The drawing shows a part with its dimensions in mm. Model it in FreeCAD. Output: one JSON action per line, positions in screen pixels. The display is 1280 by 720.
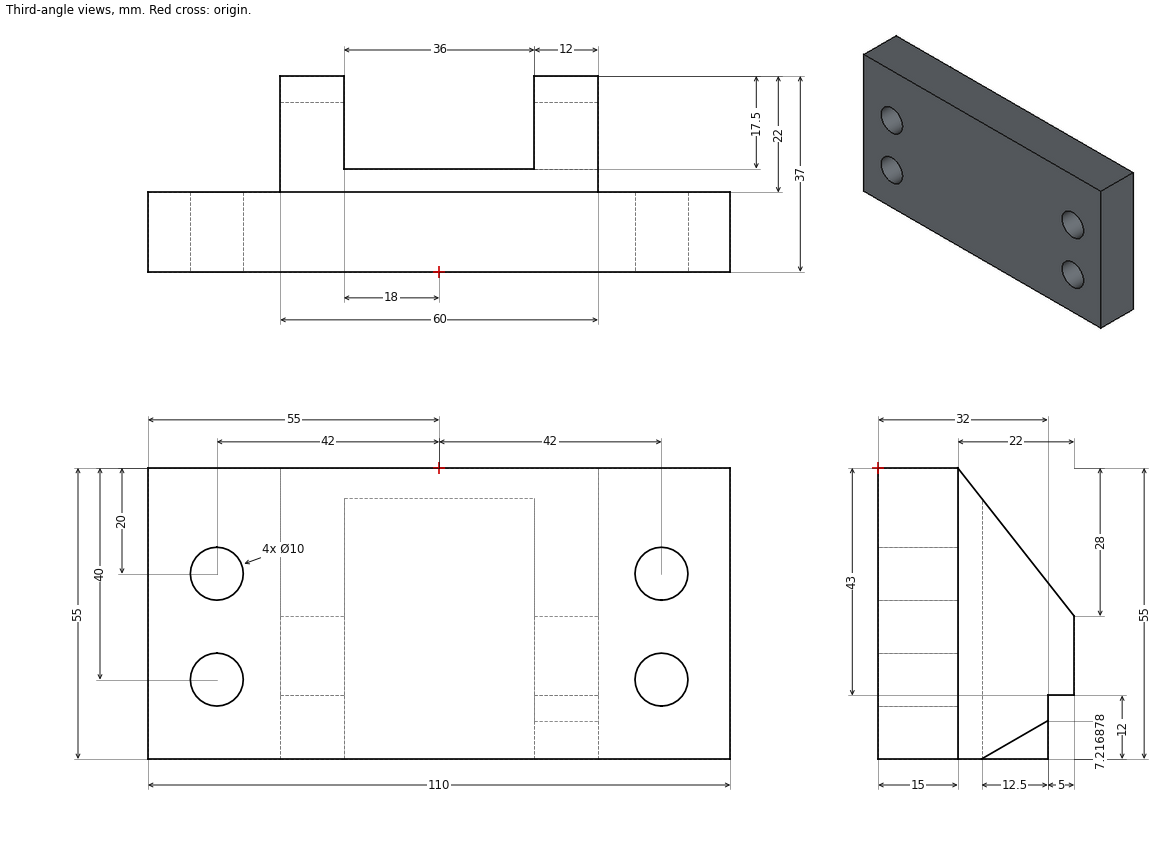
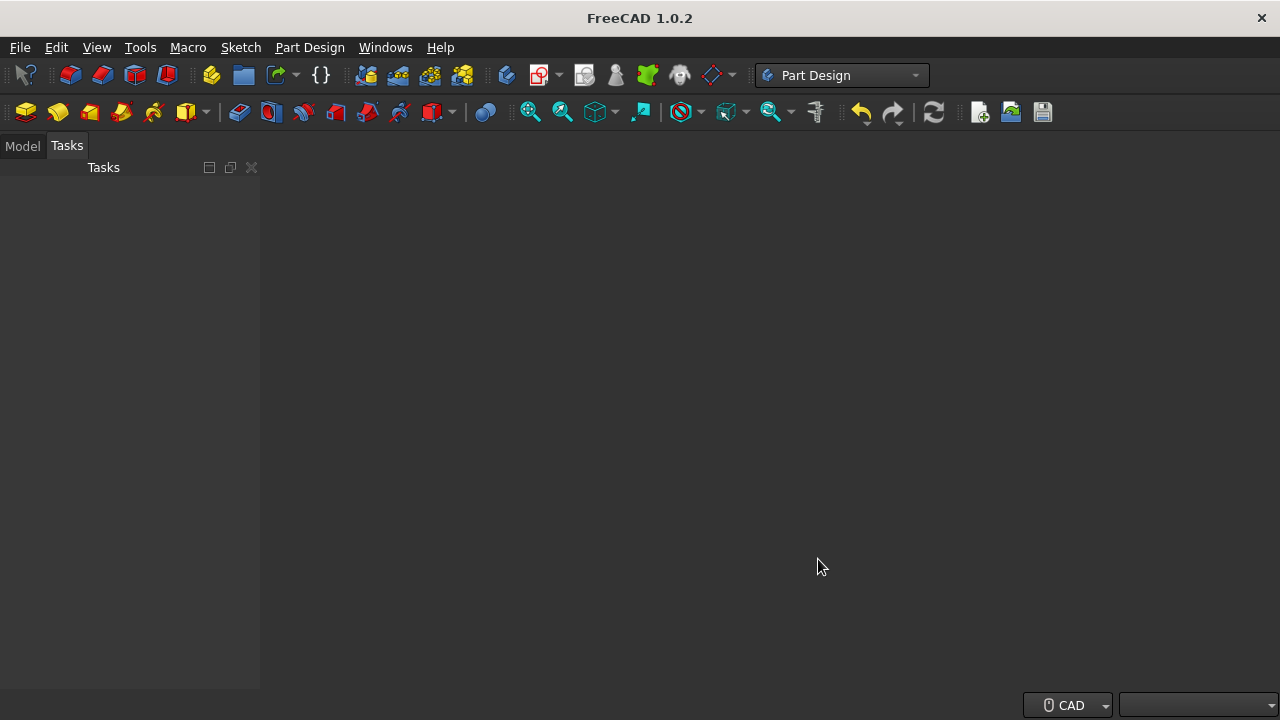
{"action": "left_click", "coordinate": [980, 112]}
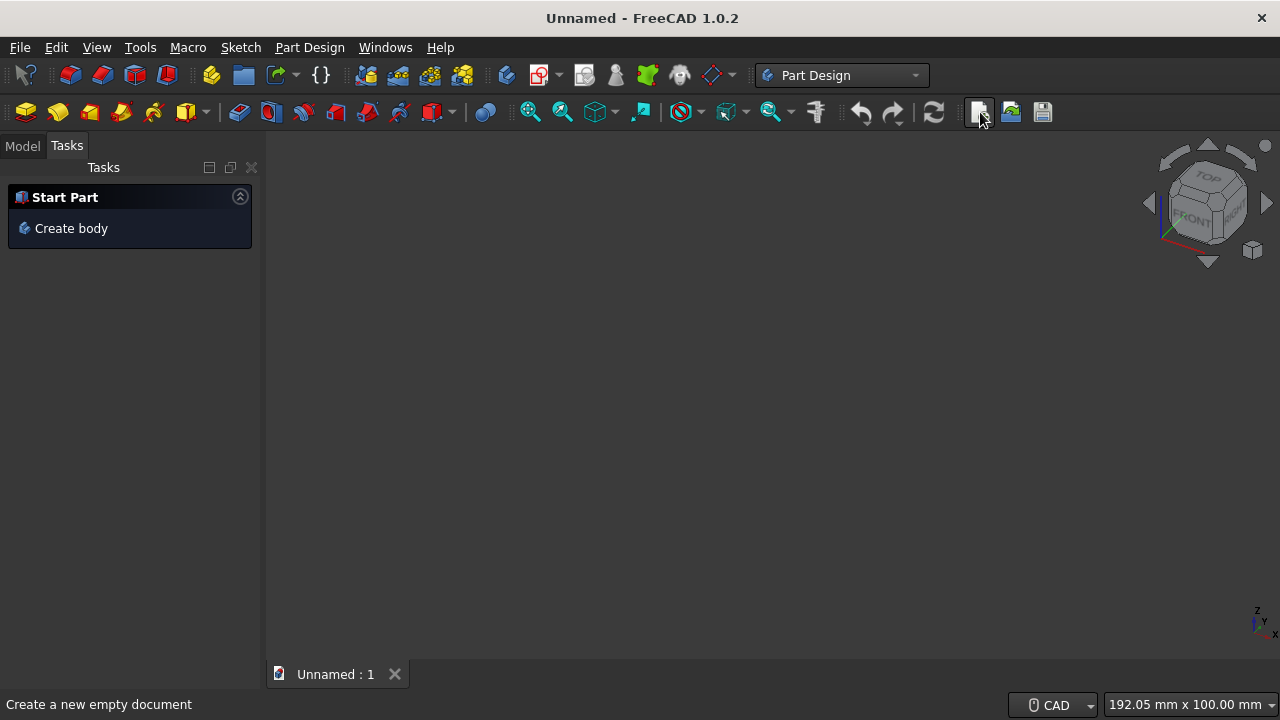
{"action": "left_click", "coordinate": [540, 76]}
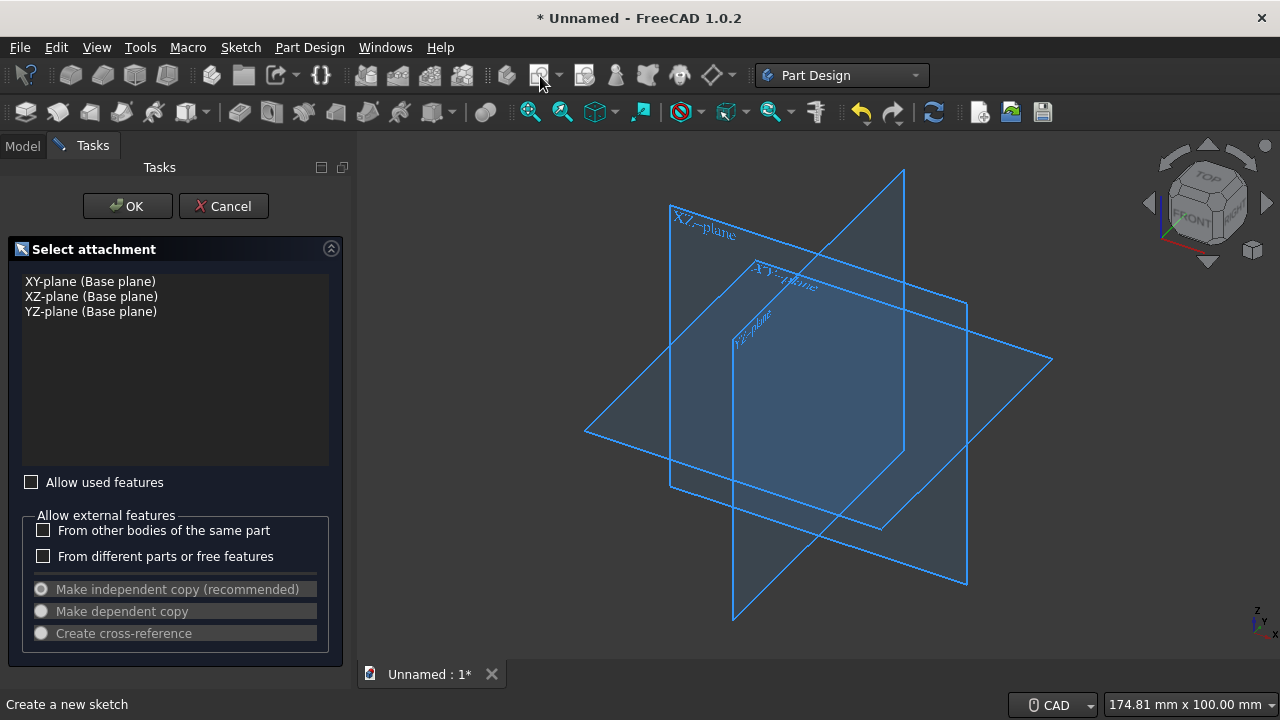
{"action": "left_click", "coordinate": [82, 296]}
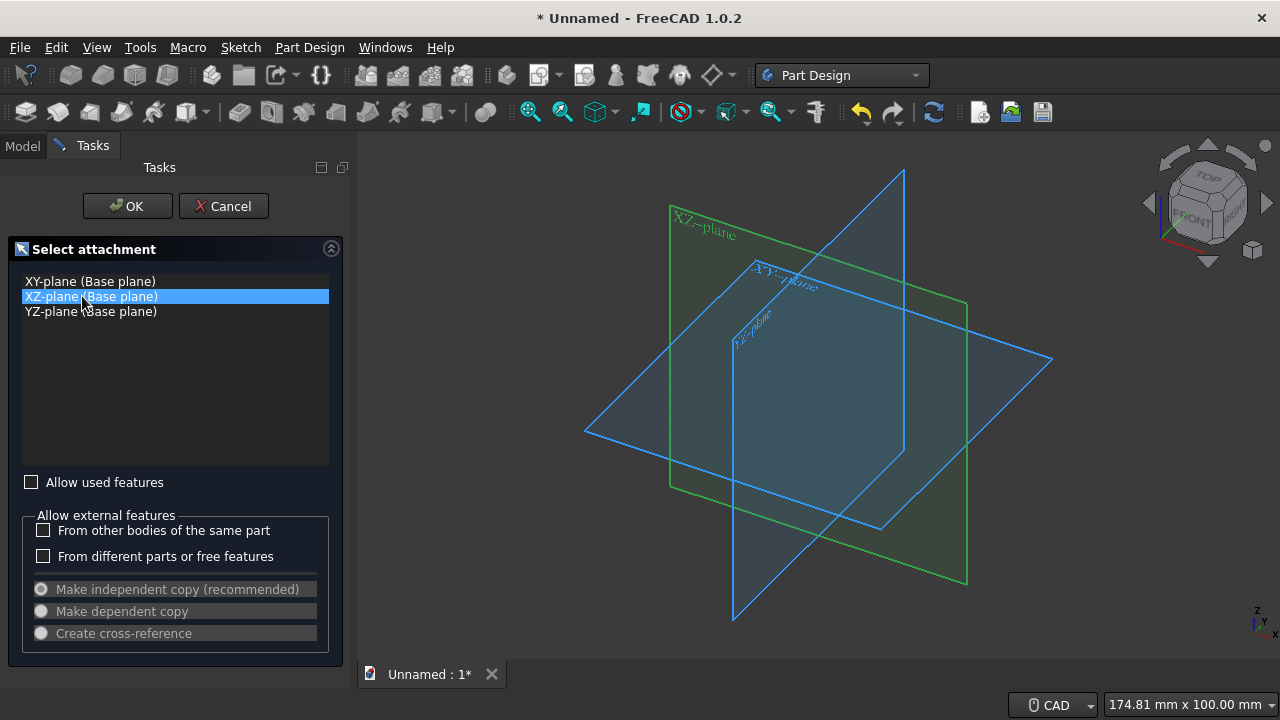
{"action": "left_click", "coordinate": [128, 206]}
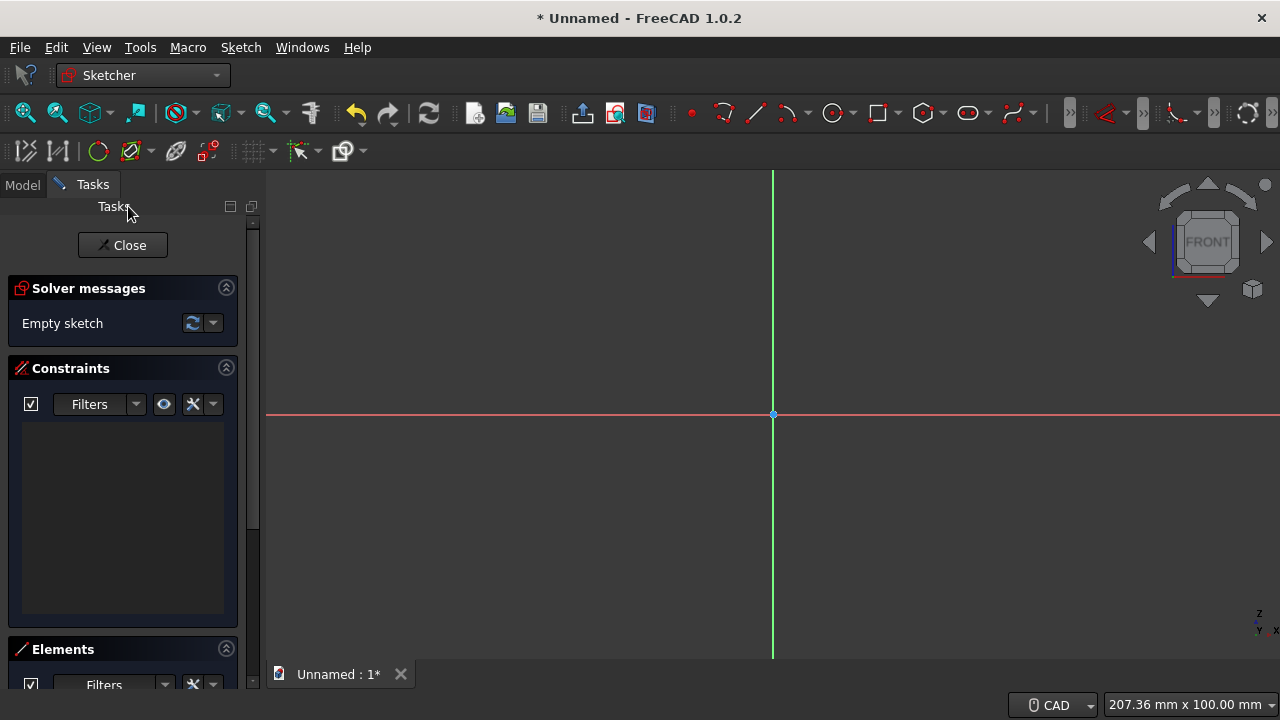
{"action": "scroll", "coordinate": [395, 198], "scroll_direction": "down", "scroll_amount": 1}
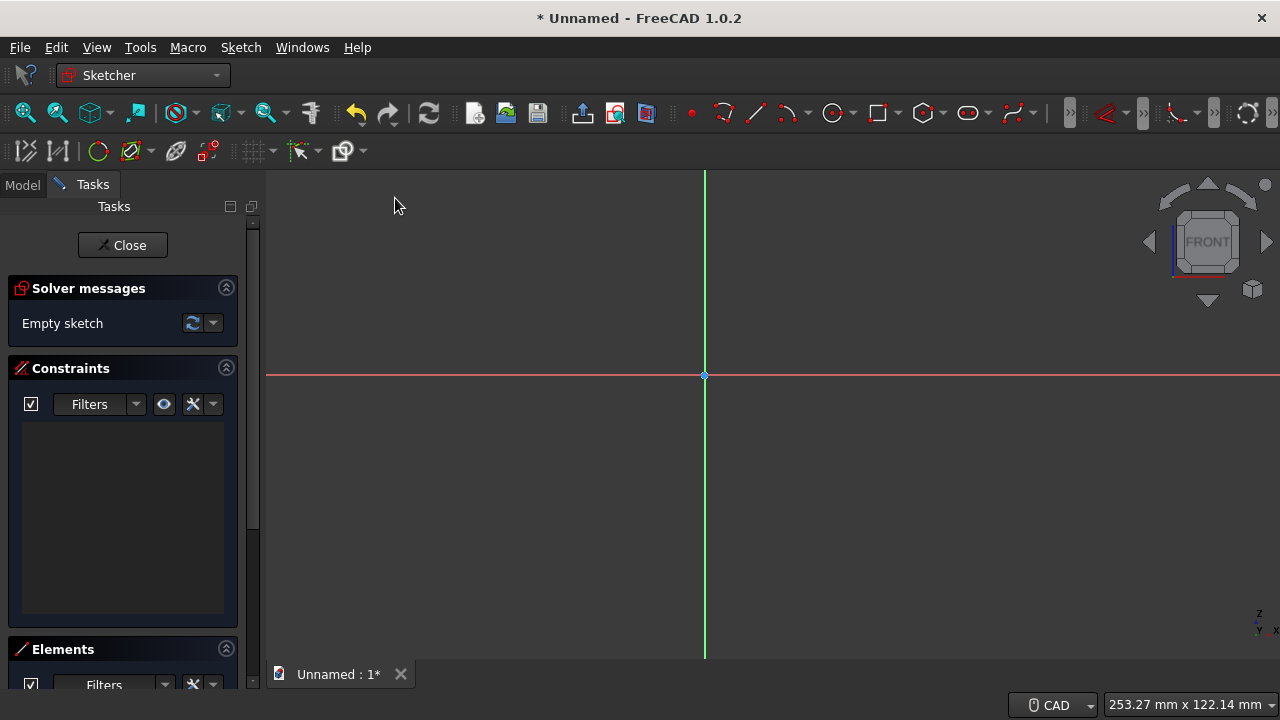
{"action": "left_click", "coordinate": [878, 114]}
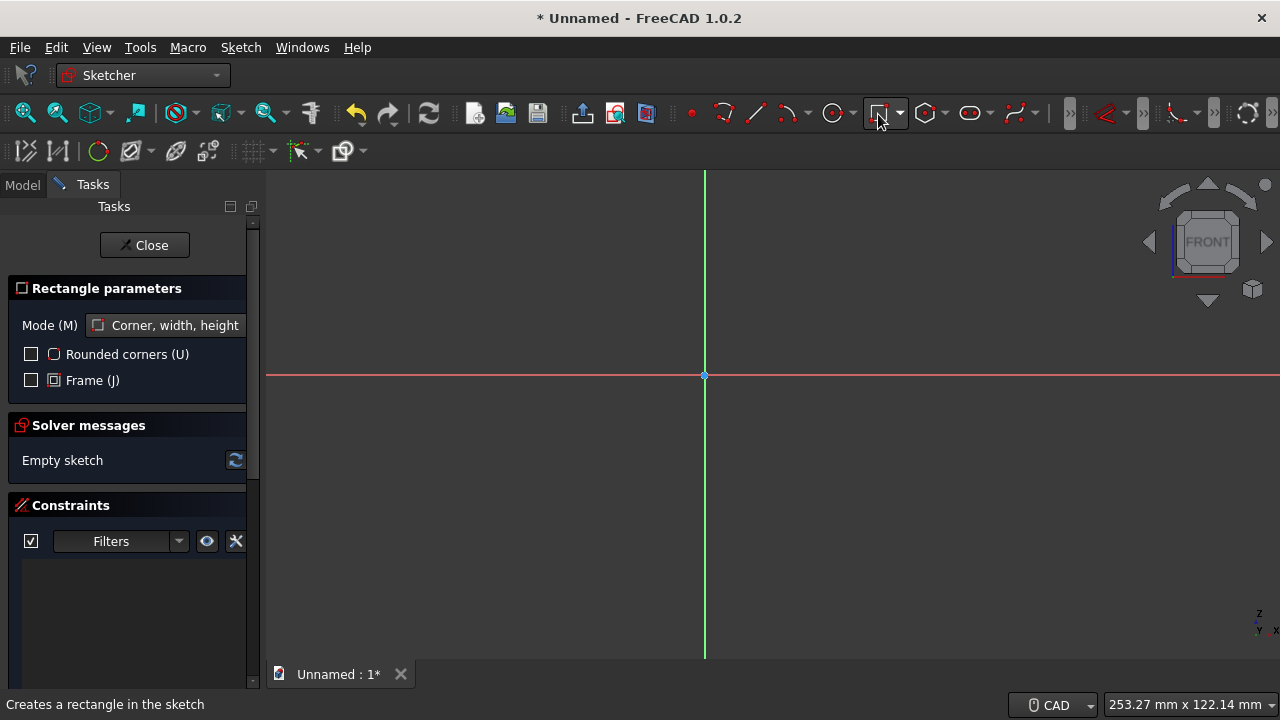
{"action": "left_click", "coordinate": [484, 375]}
{"action": "left_click", "coordinate": [925, 595]}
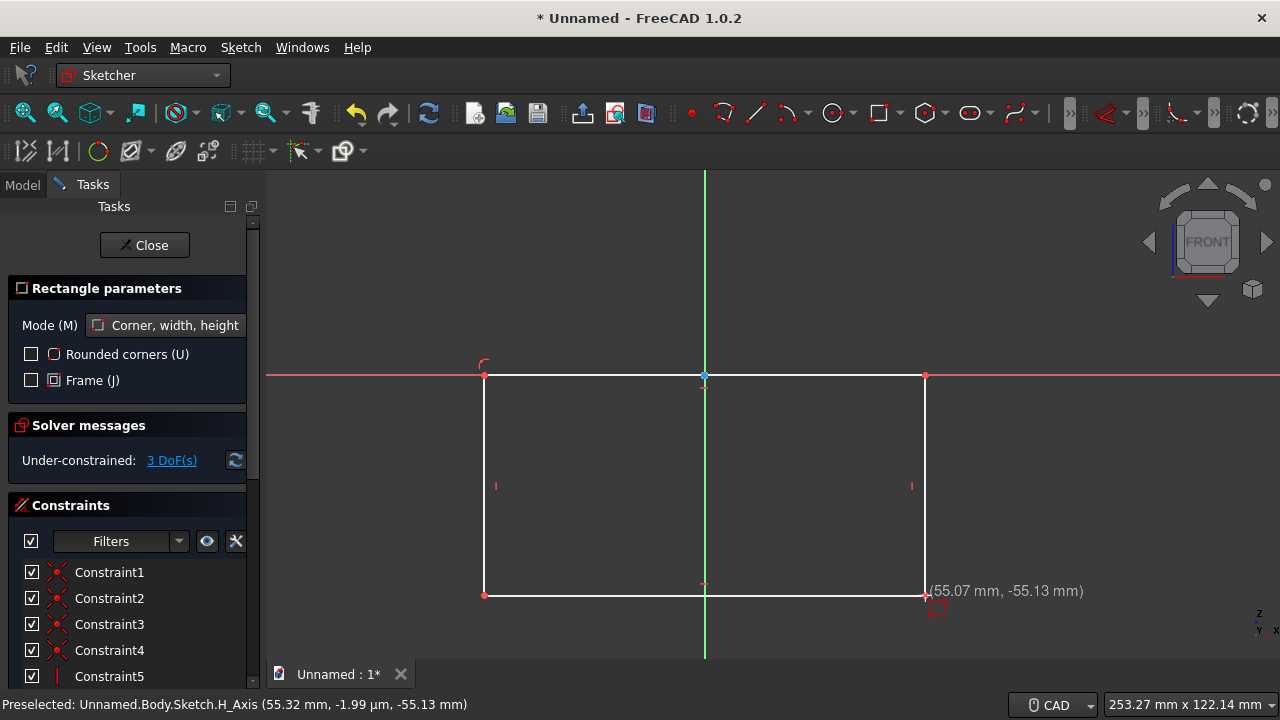
{"action": "left_click", "coordinate": [834, 114]}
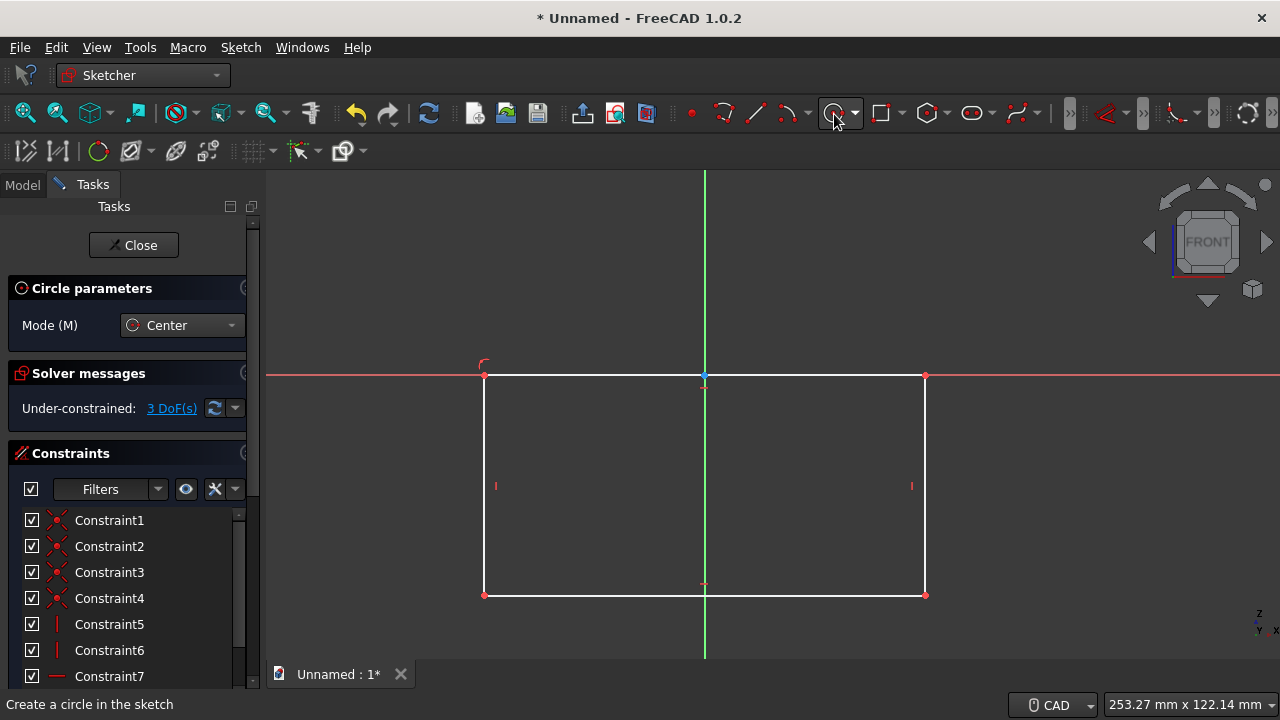
{"action": "left_click", "coordinate": [536, 455]}
{"action": "left_click", "coordinate": [551, 441]}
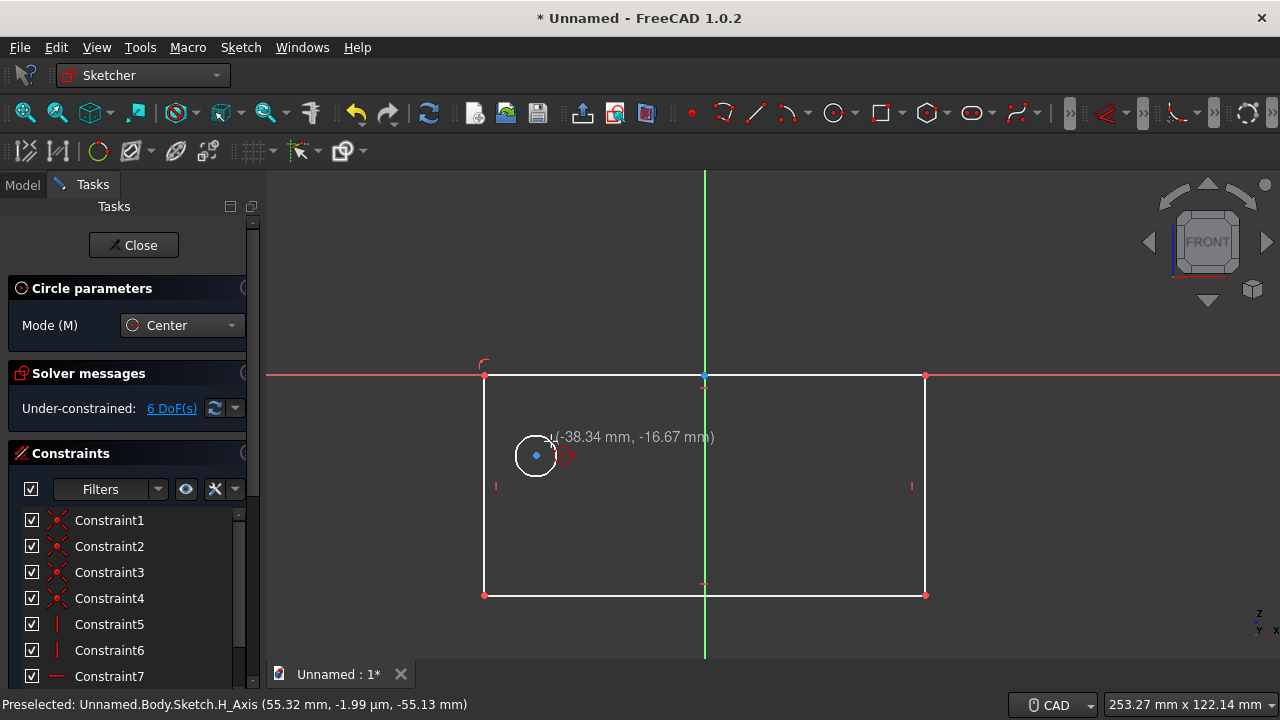
{"action": "left_click", "coordinate": [873, 455]}
{"action": "left_click", "coordinate": [887, 441]}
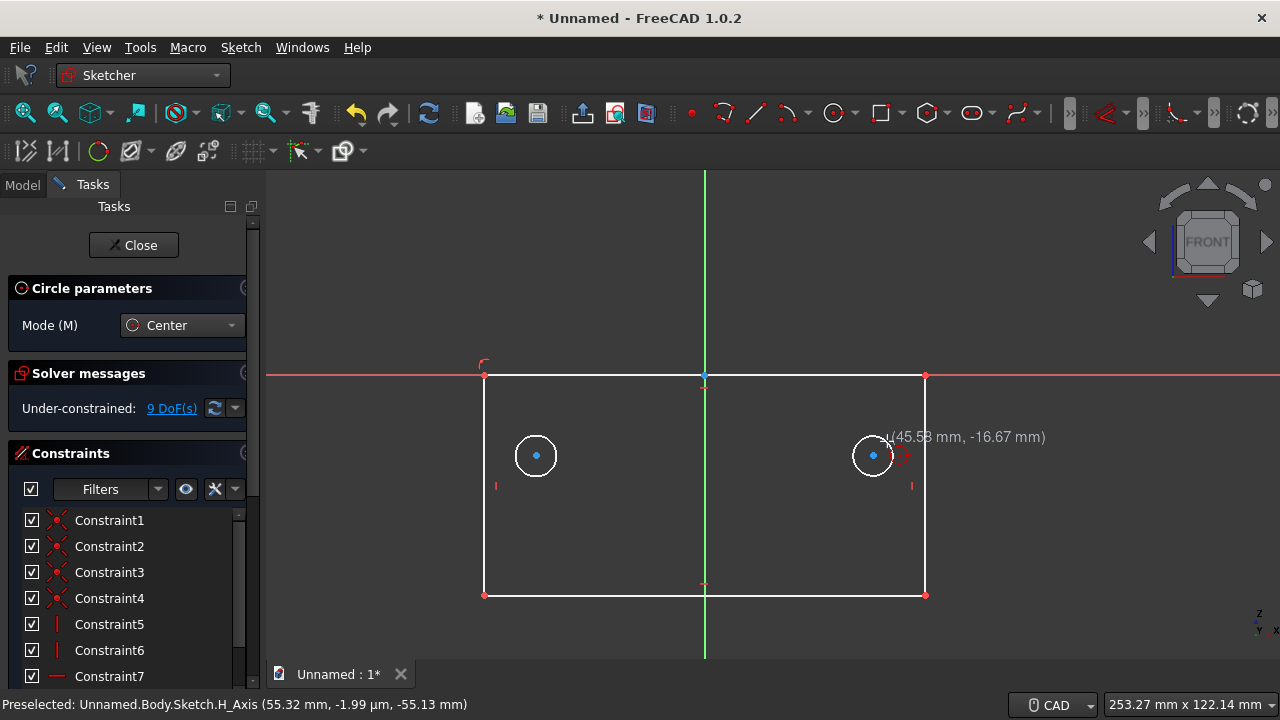
{"action": "left_click", "coordinate": [536, 535]}
{"action": "left_click", "coordinate": [551, 521]}